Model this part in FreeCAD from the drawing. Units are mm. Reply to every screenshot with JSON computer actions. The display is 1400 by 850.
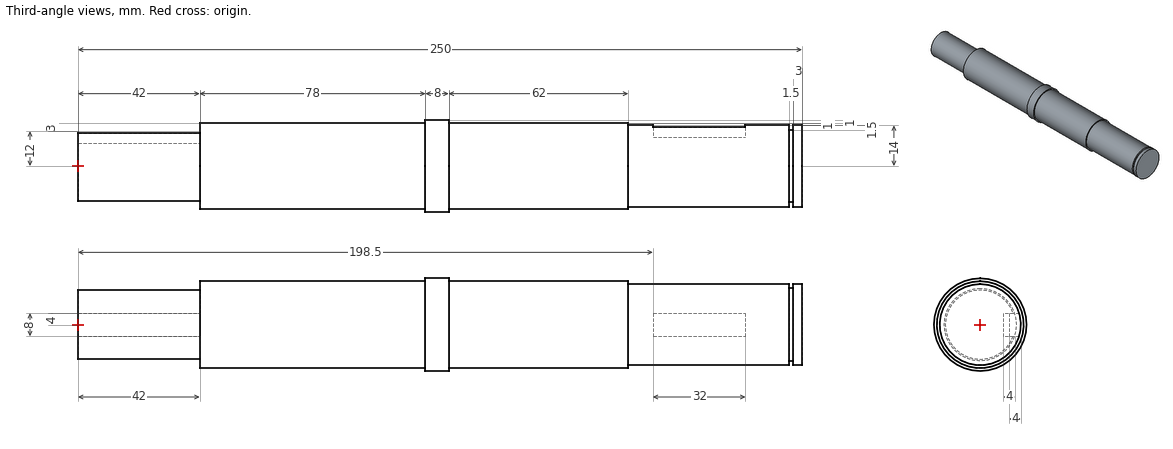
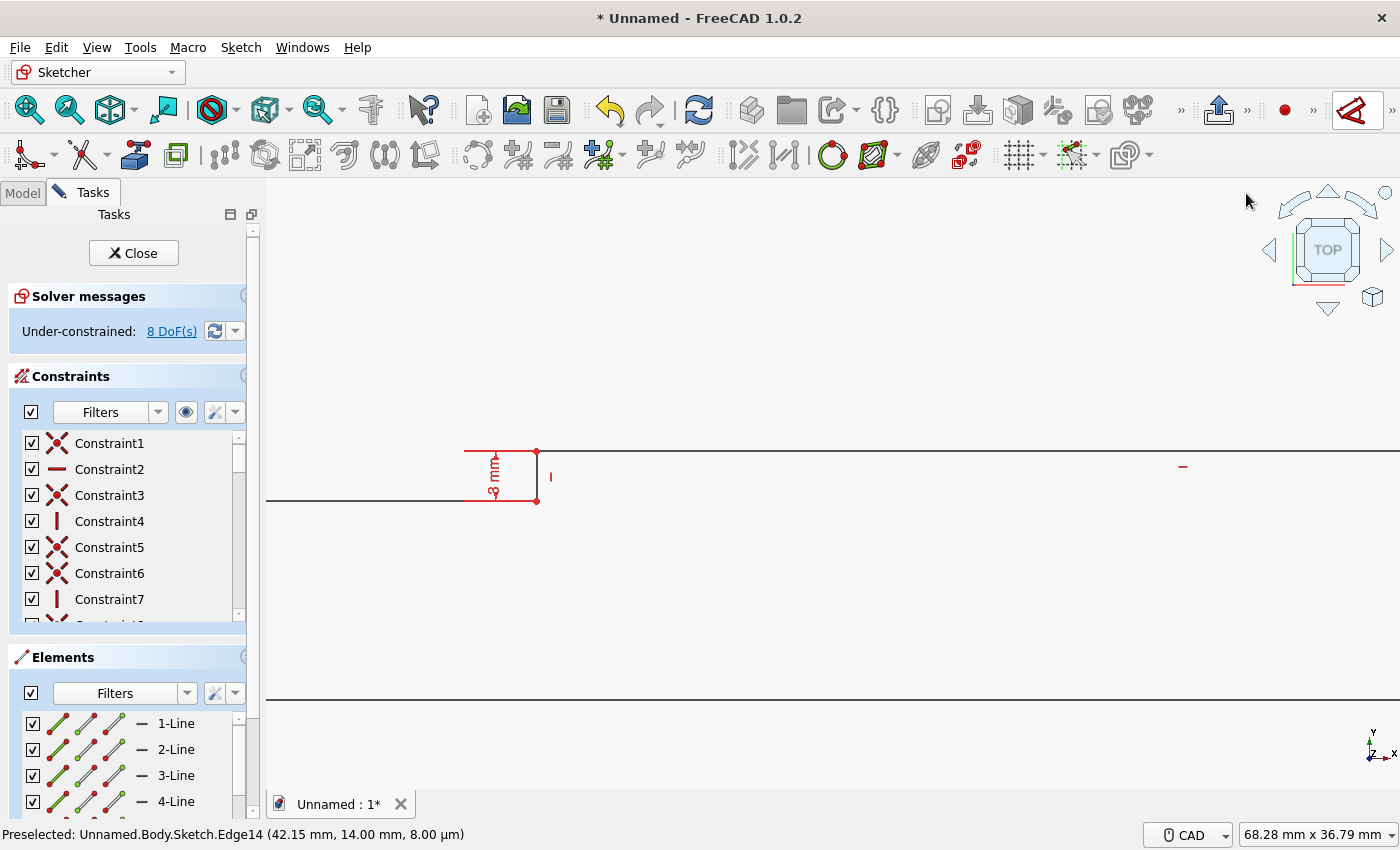
{"action": "scroll", "coordinate": [537, 467], "scroll_direction": "down", "scroll_amount": 9}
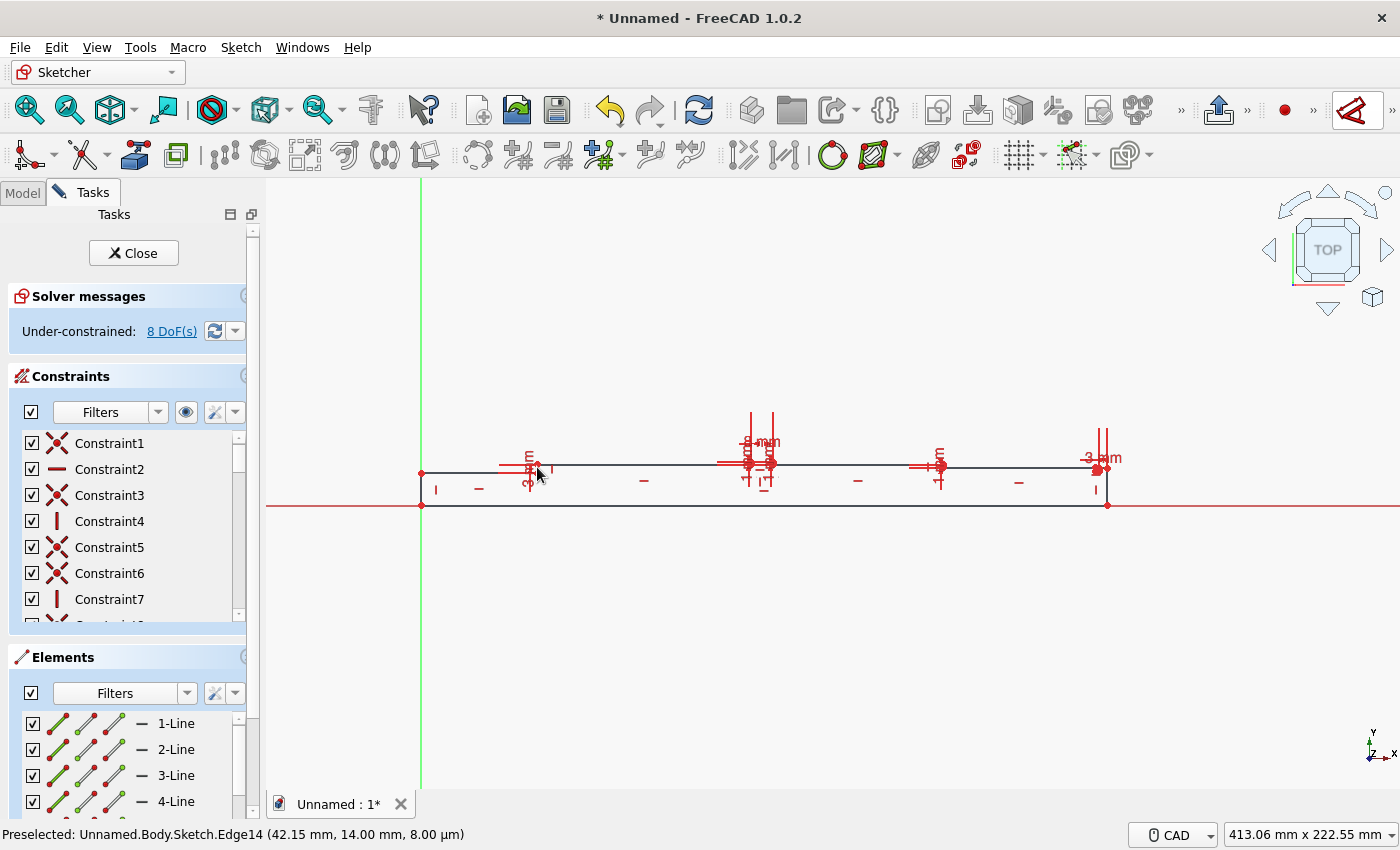
{"action": "left_click", "coordinate": [1107, 498]}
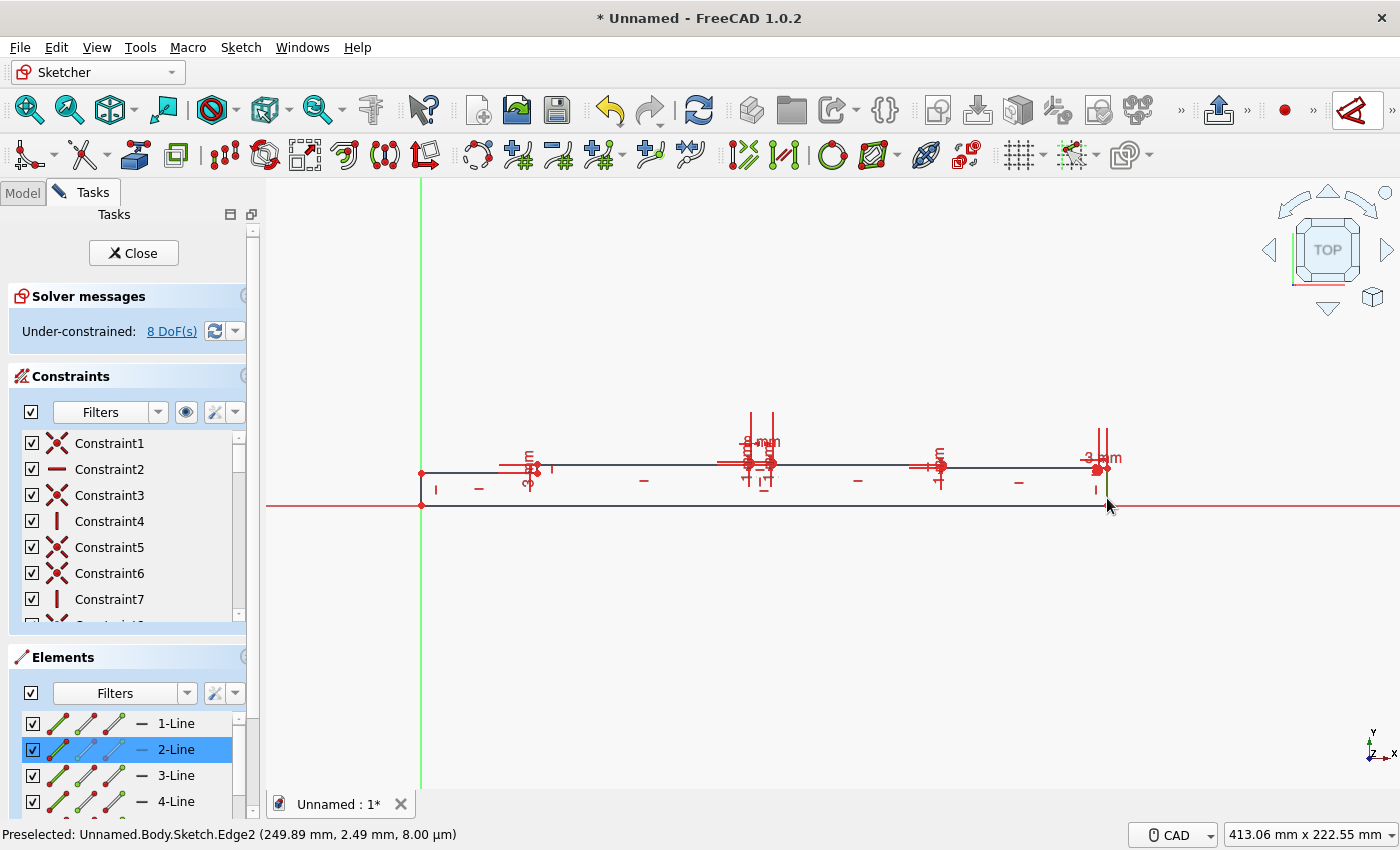
{"action": "key", "text": "i"}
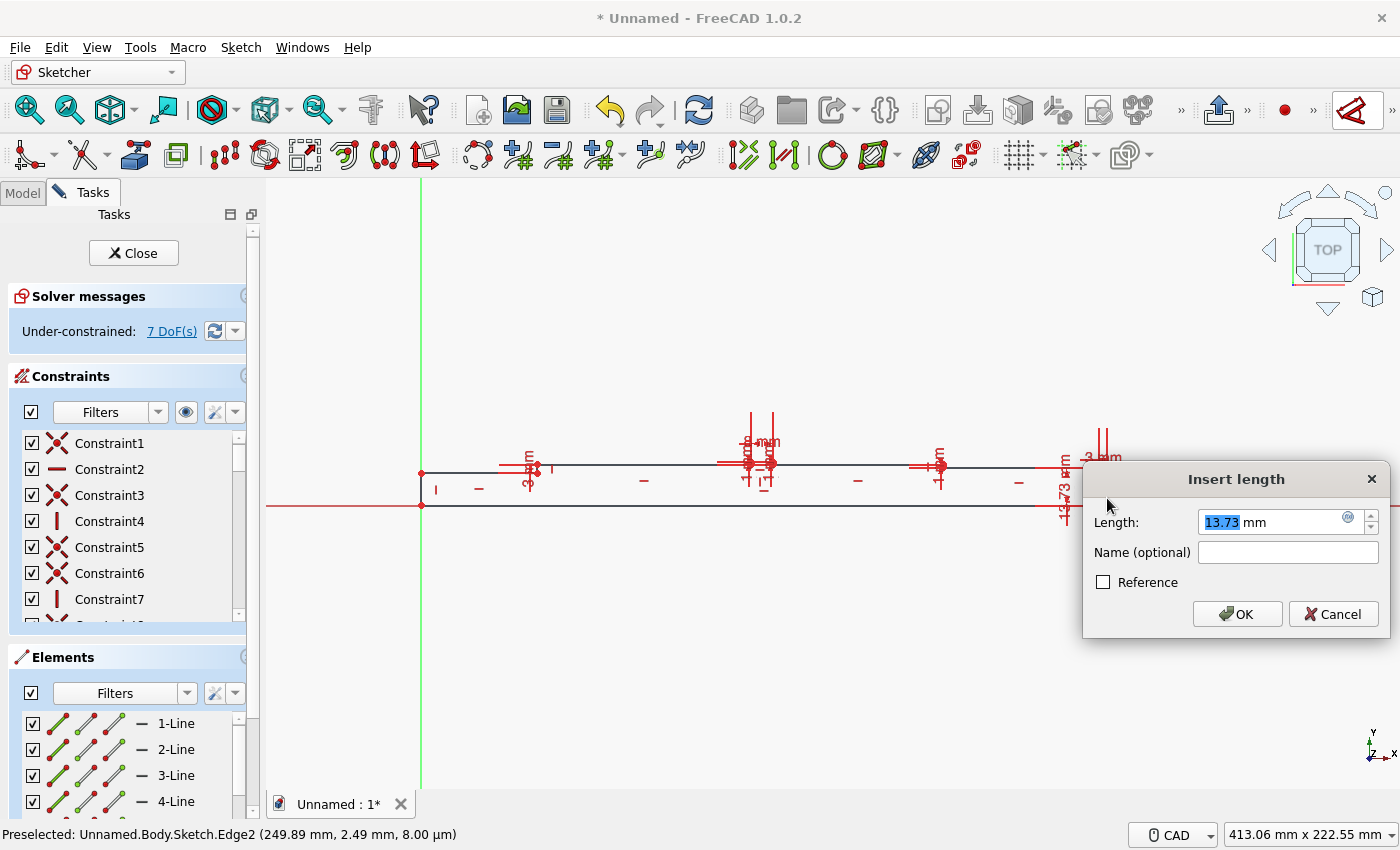
{"action": "type", "text": "14"}
{"action": "key", "text": "Return"}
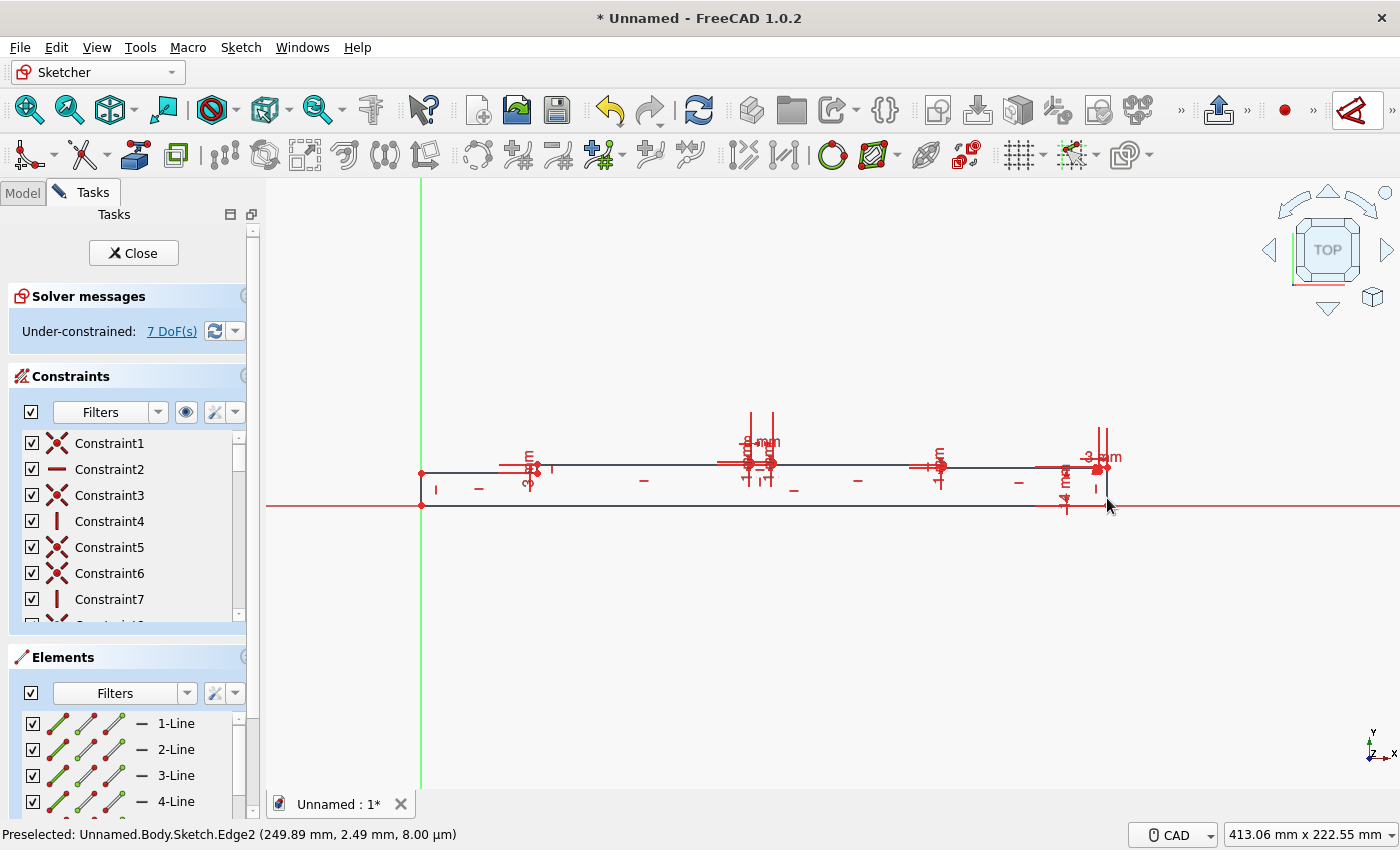
{"action": "left_click", "coordinate": [892, 465]}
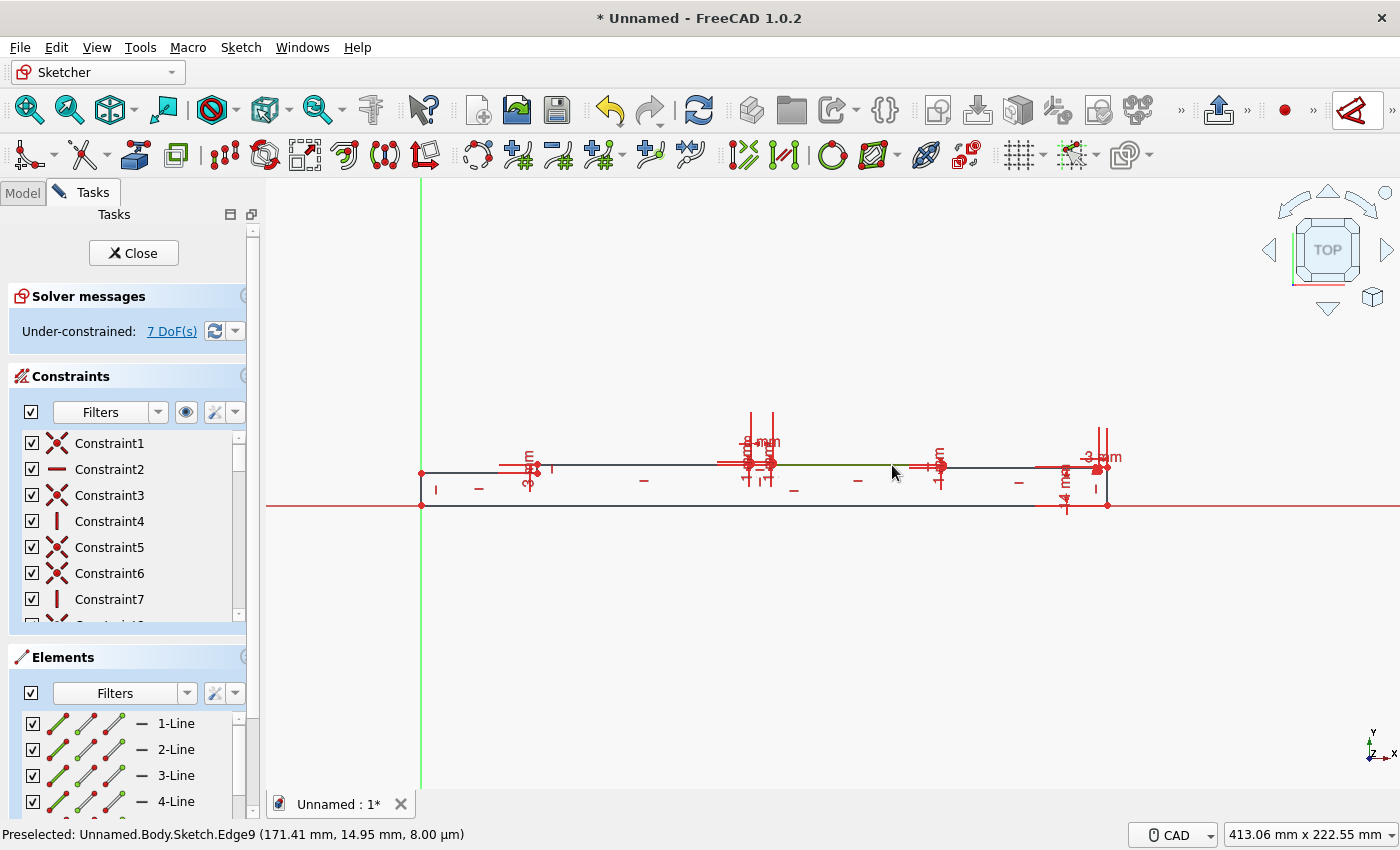
{"action": "left_click", "coordinate": [1378, 110]}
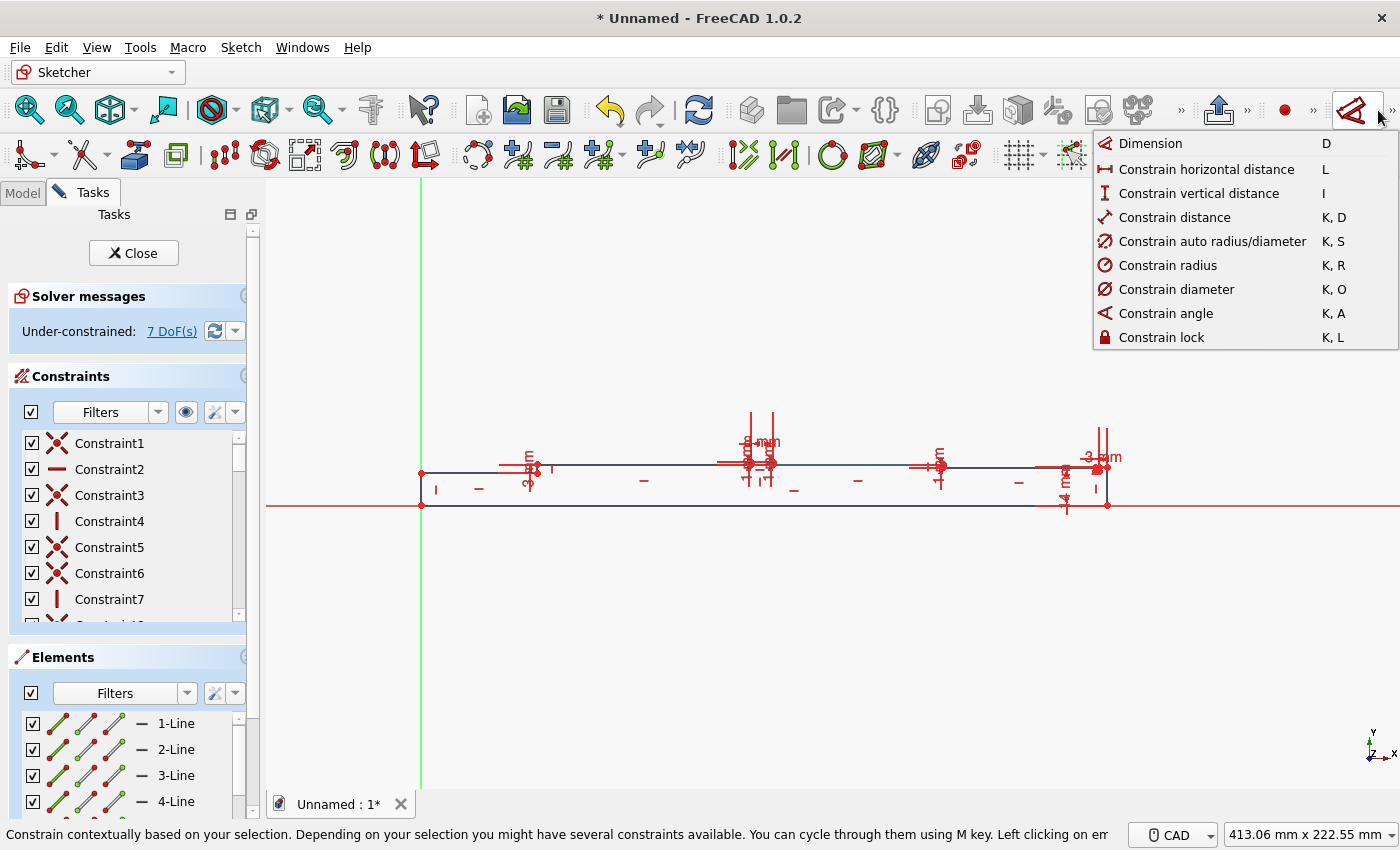
{"action": "left_click", "coordinate": [1246, 169]}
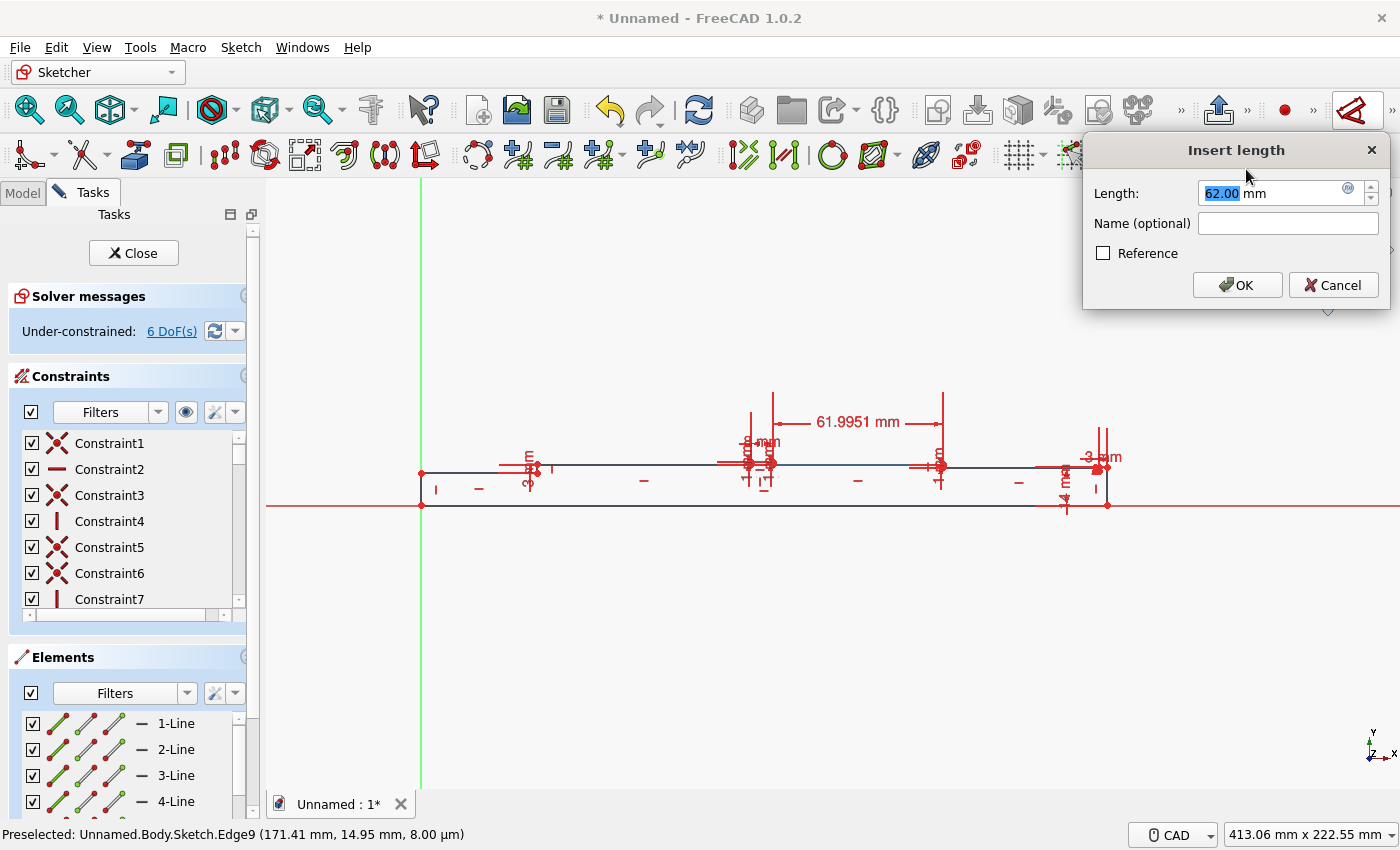
{"action": "type", "text": "62"}
{"action": "key", "text": "Return"}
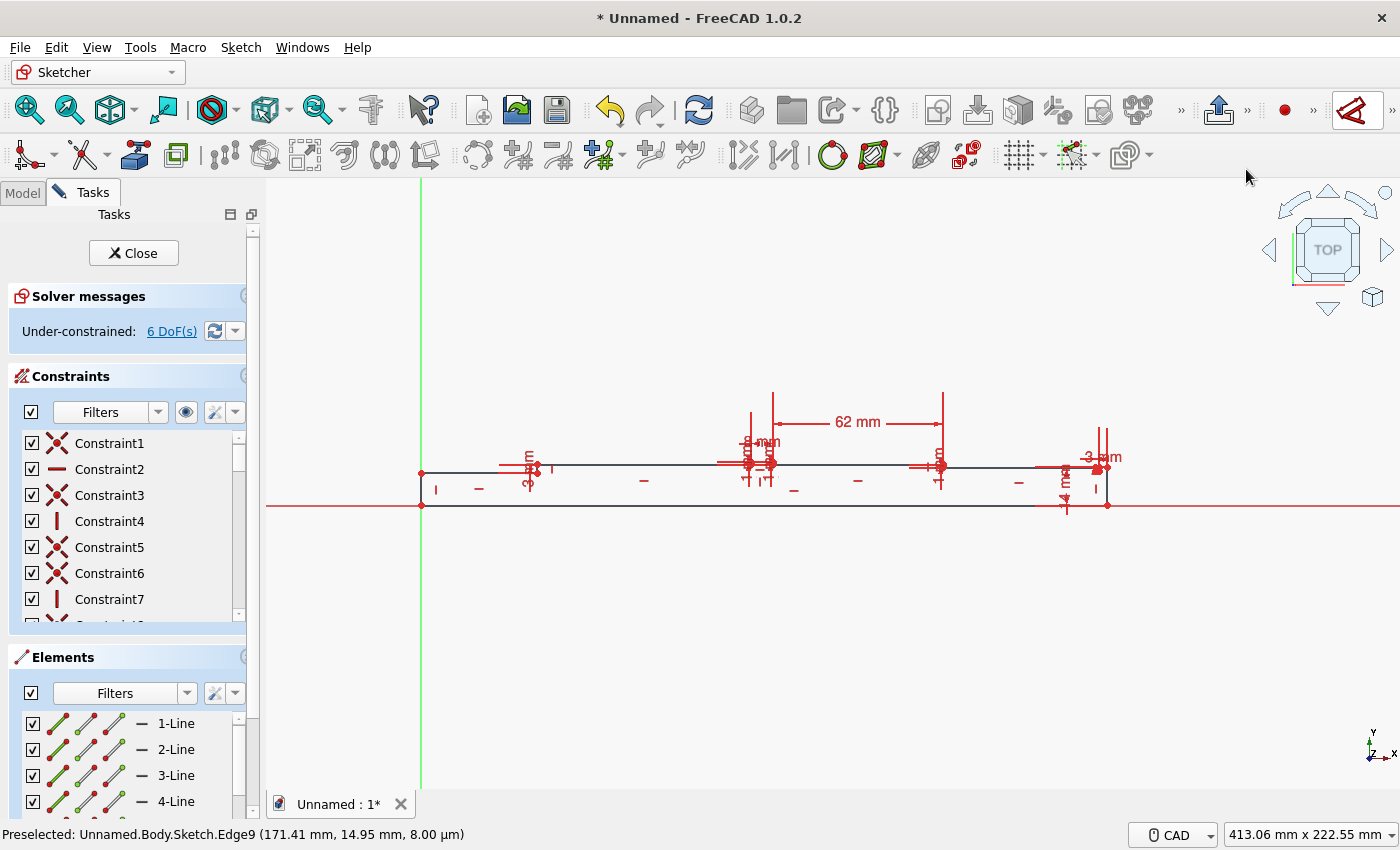
{"action": "left_click", "coordinate": [687, 465]}